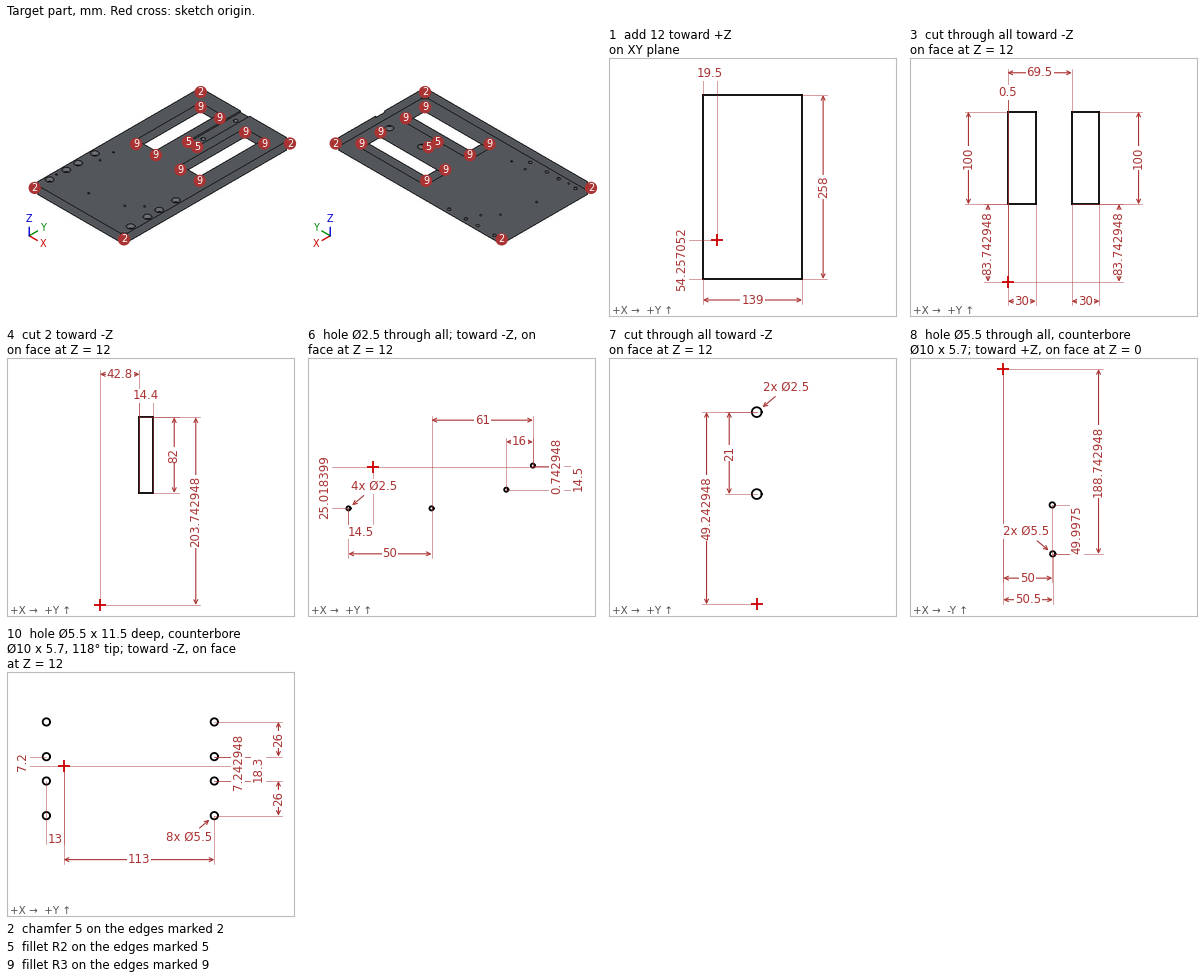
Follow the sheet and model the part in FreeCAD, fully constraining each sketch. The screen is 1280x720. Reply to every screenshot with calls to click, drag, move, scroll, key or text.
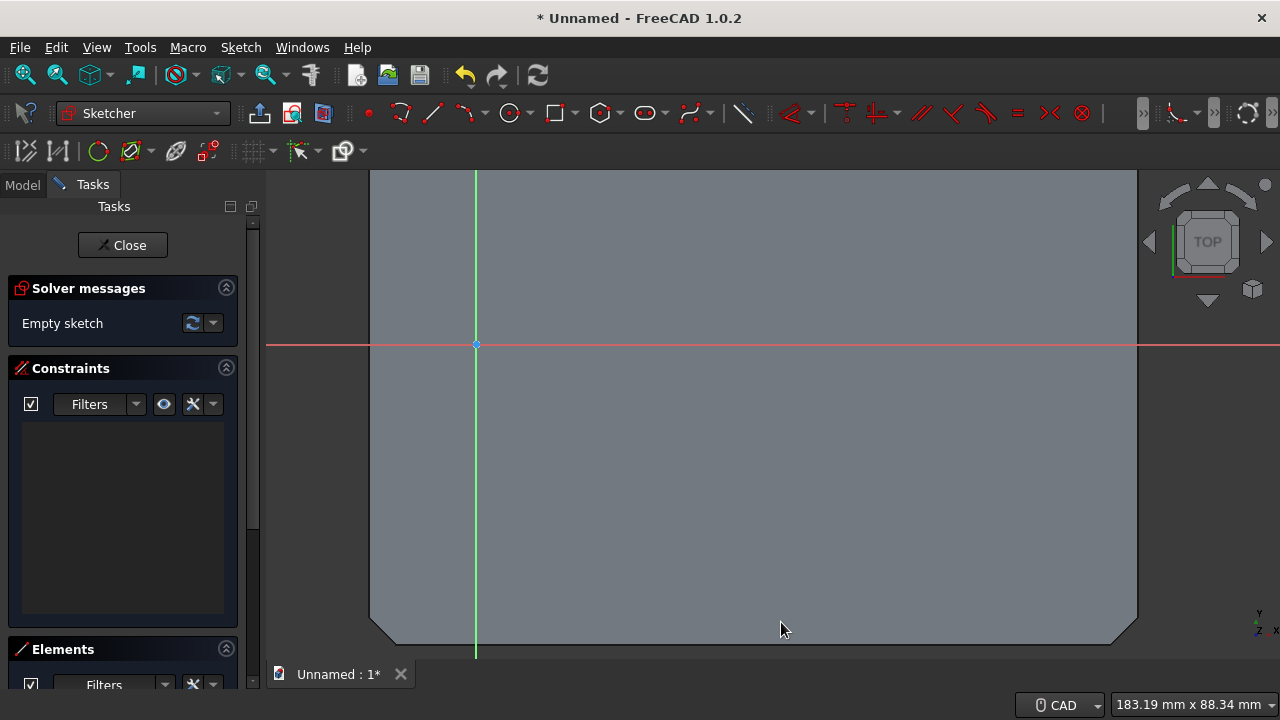
key(g)
key(c)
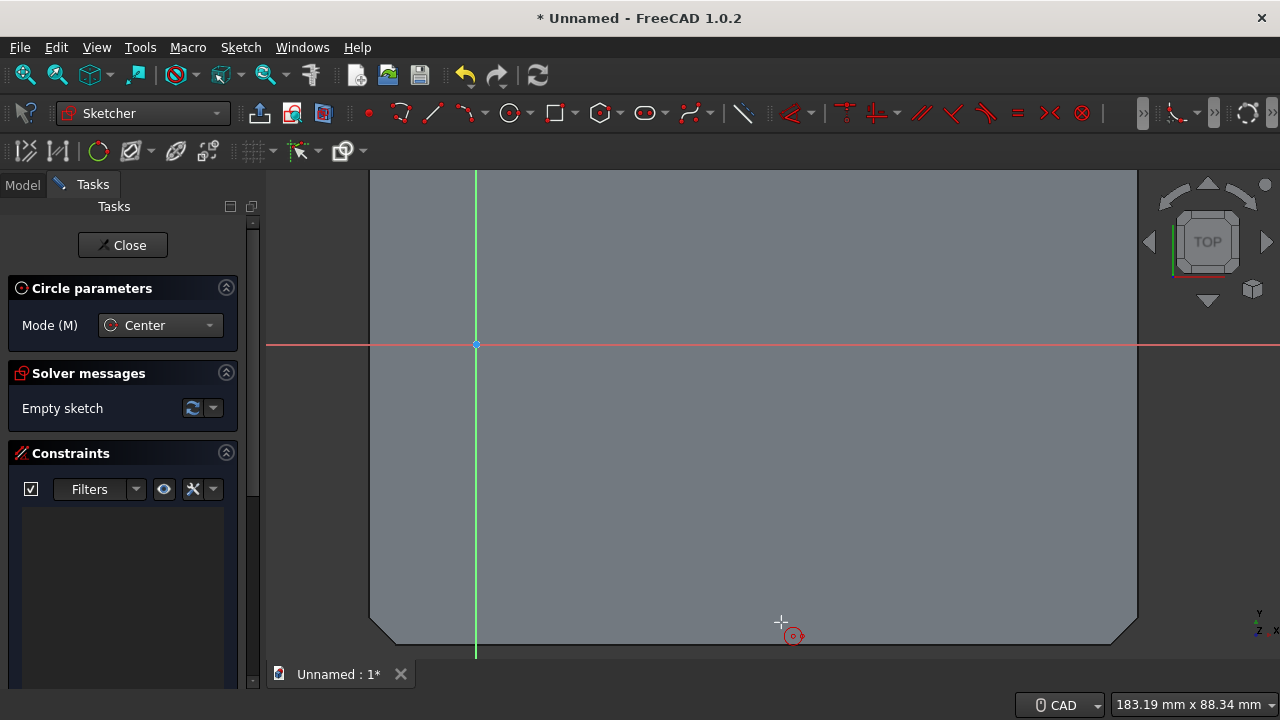
scroll(396, 483, up, 6)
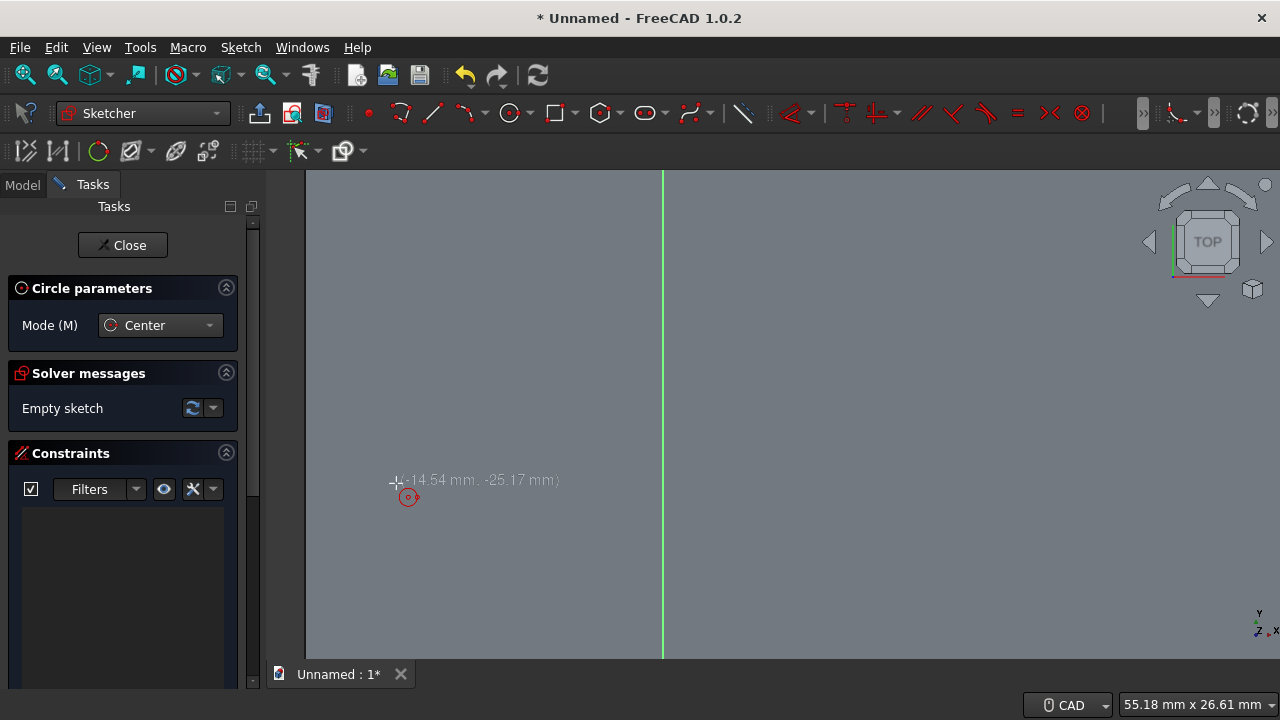
click(396, 482)
move(413, 466)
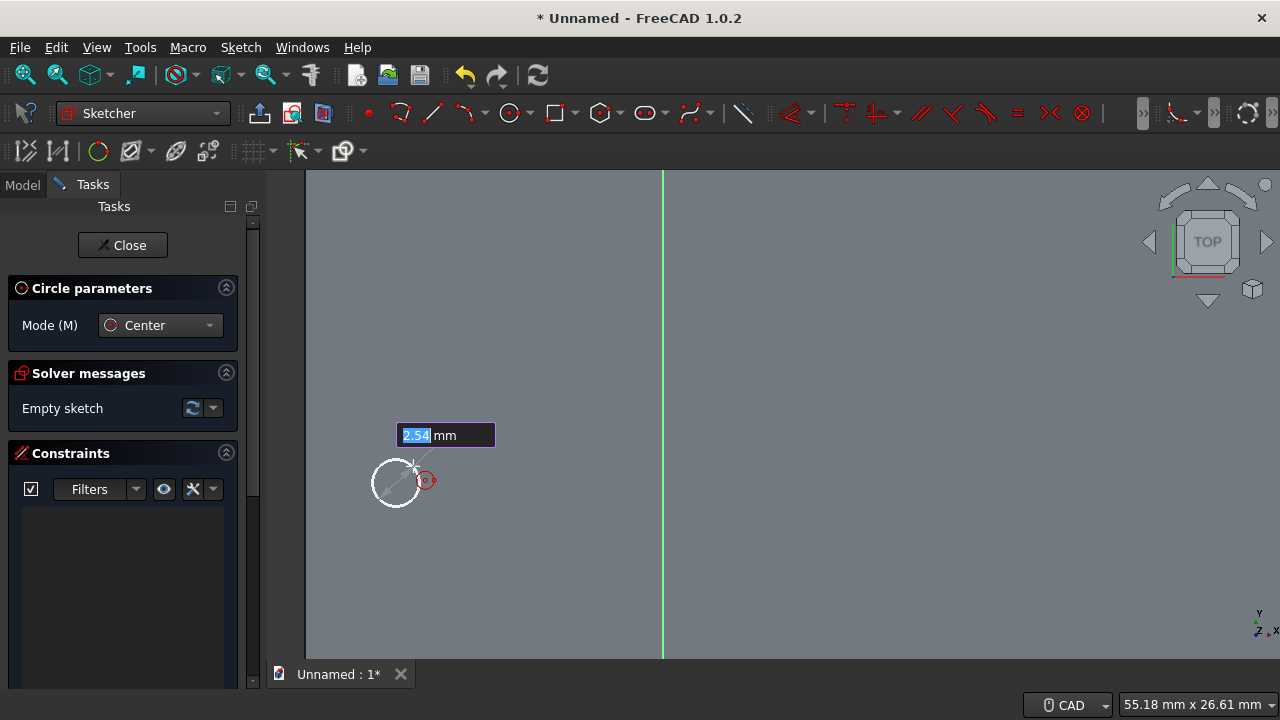
text(2.5)
key(Return)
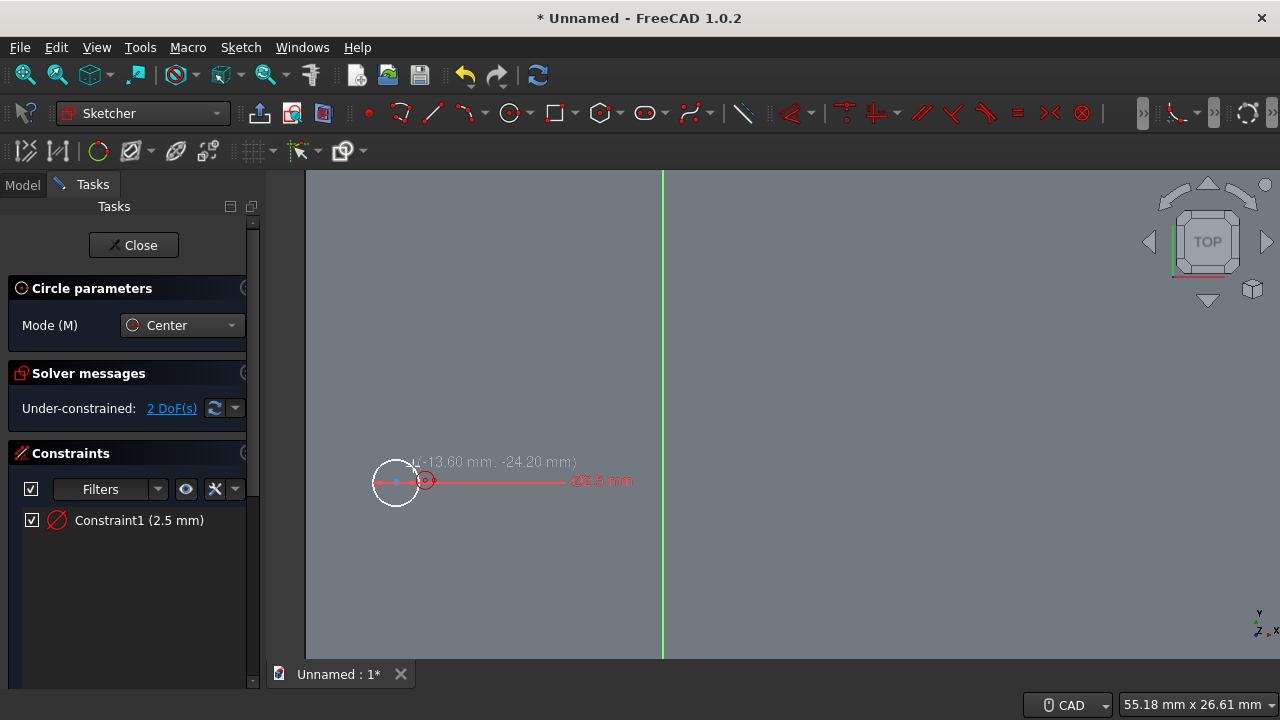
scroll(398, 487, down, 6)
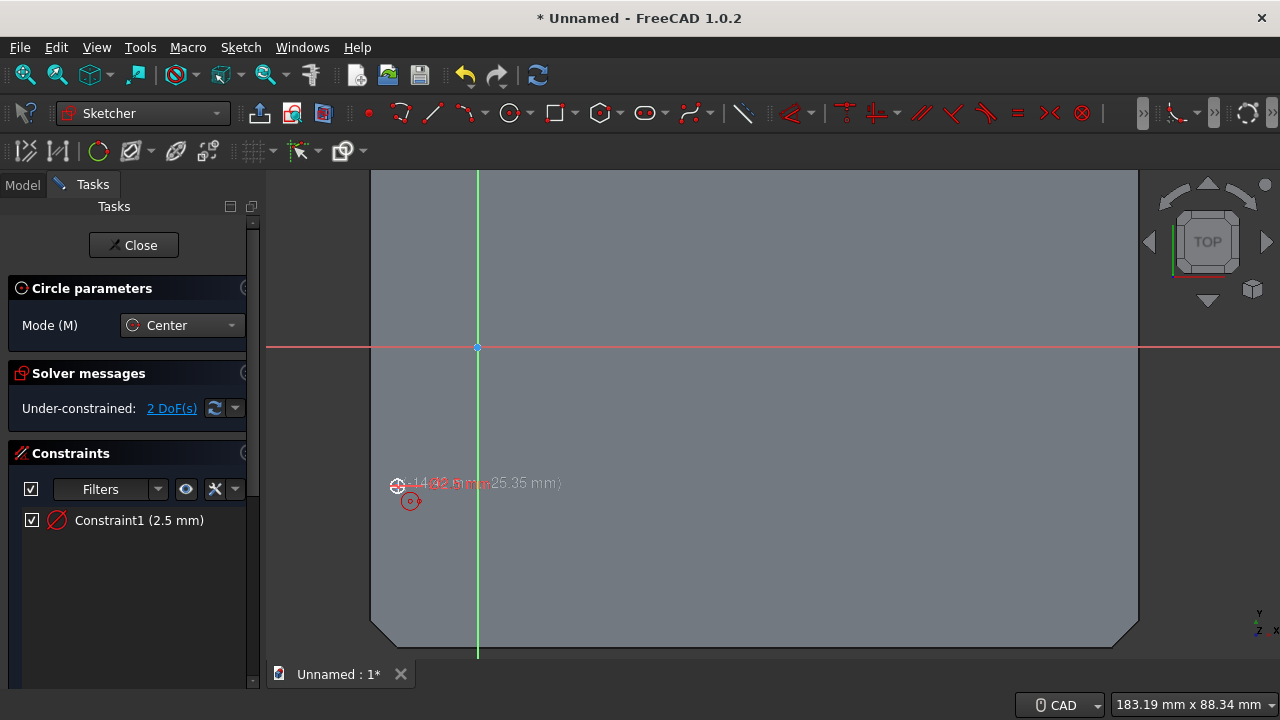
scroll(674, 486, up, 6)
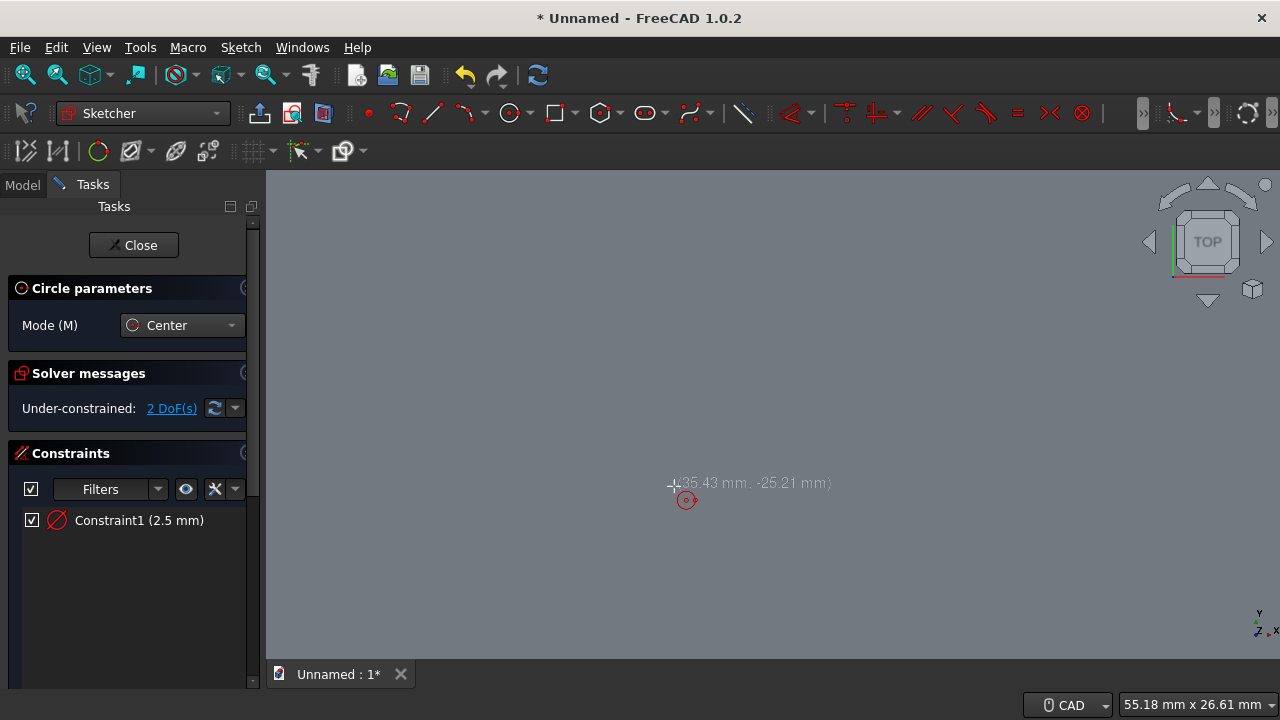
click(674, 484)
move(691, 468)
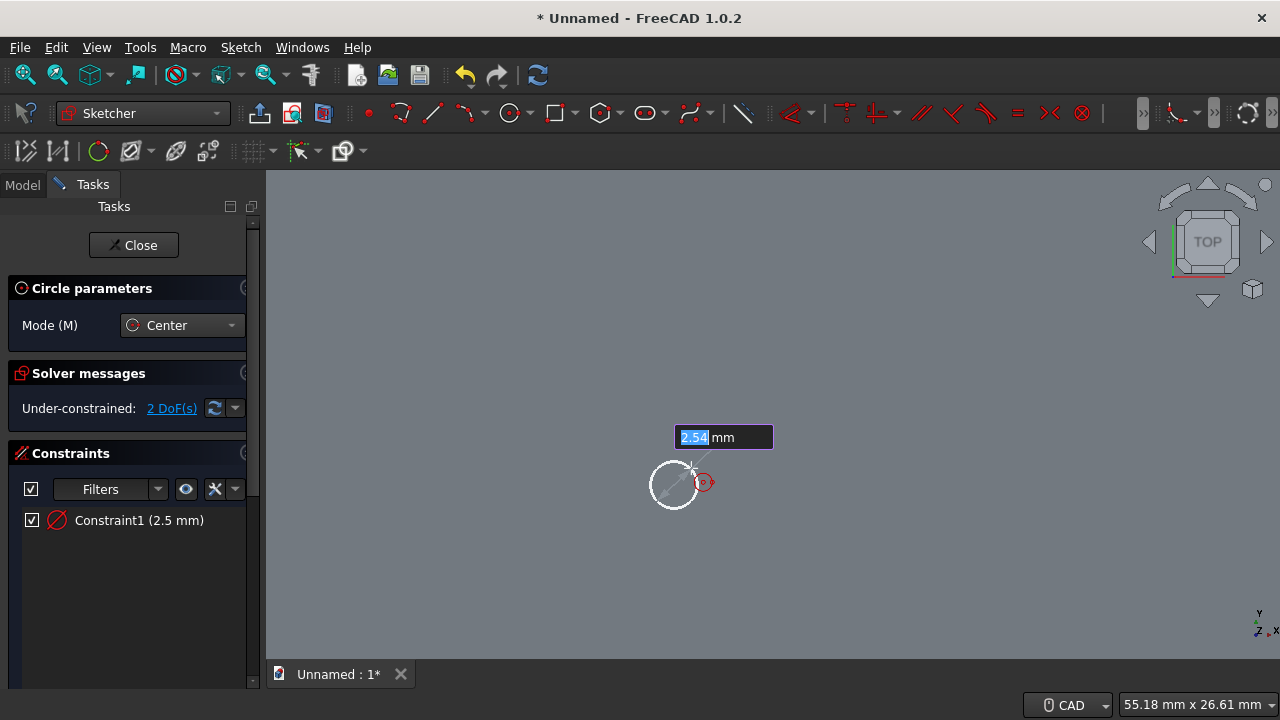
text(2.5)
key(Return)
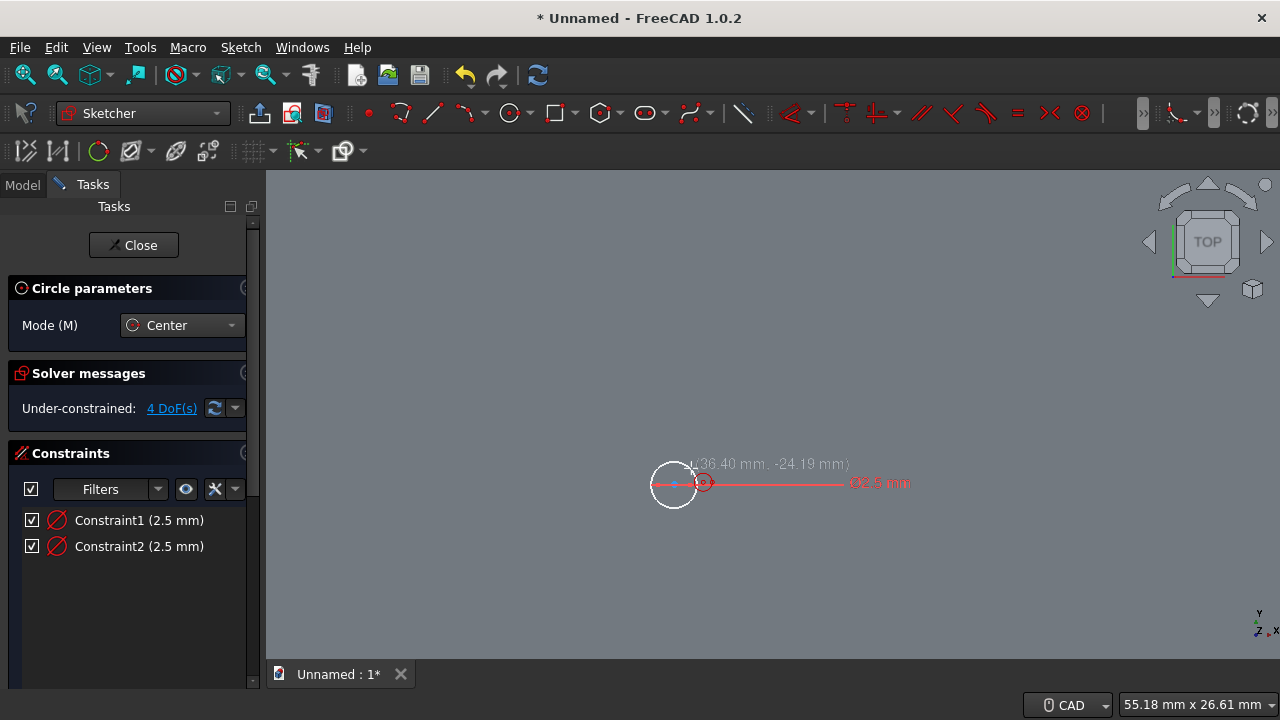
scroll(674, 486, down, 6)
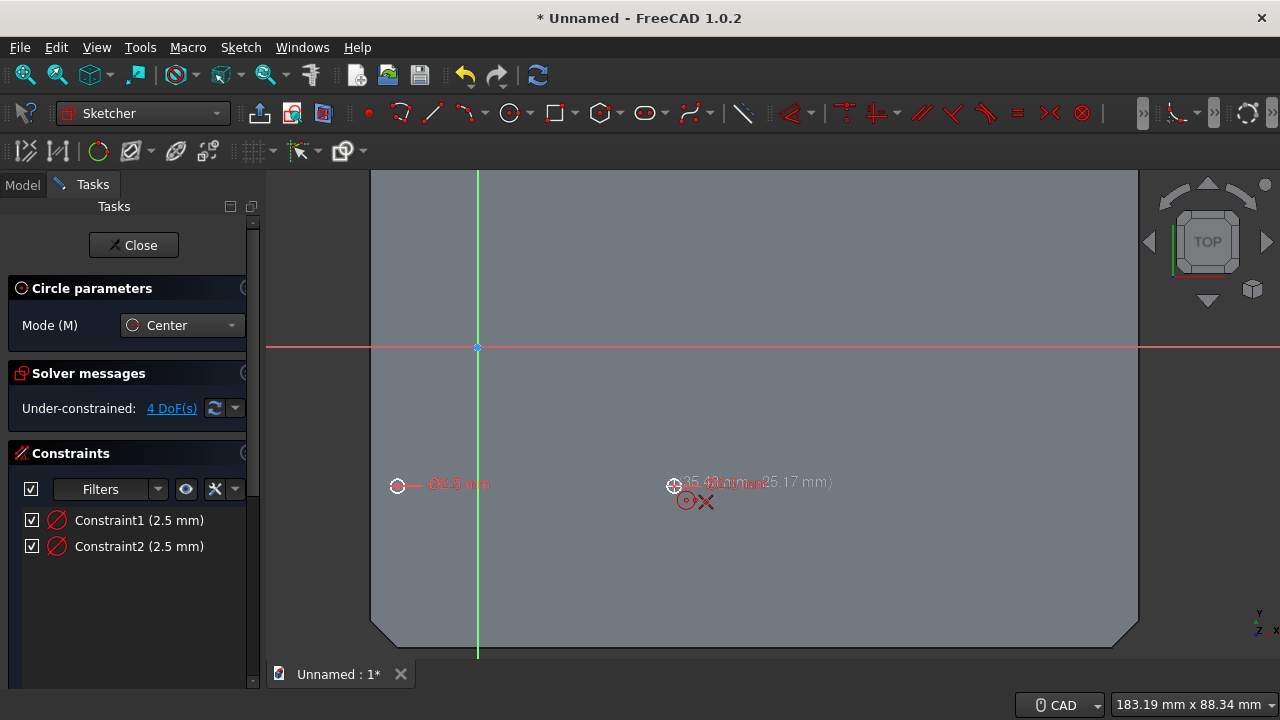
scroll(1012, 343, up, 7)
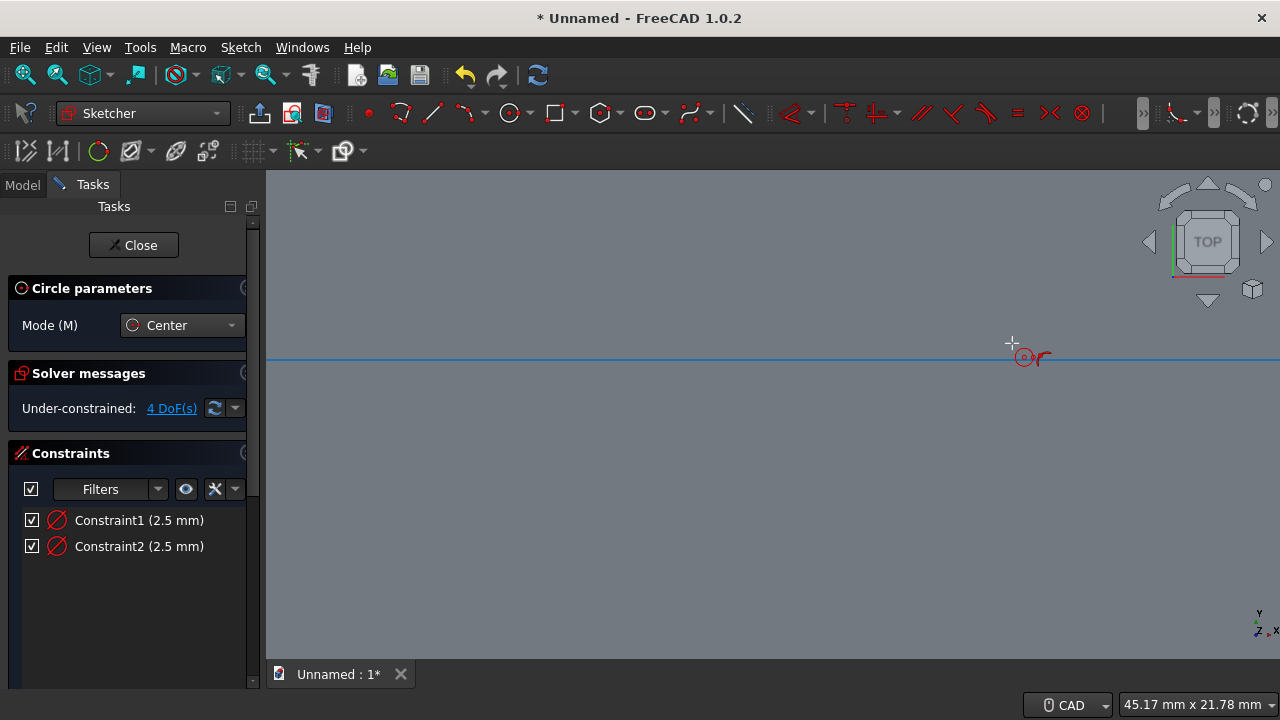
click(1010, 343)
move(1030, 323)